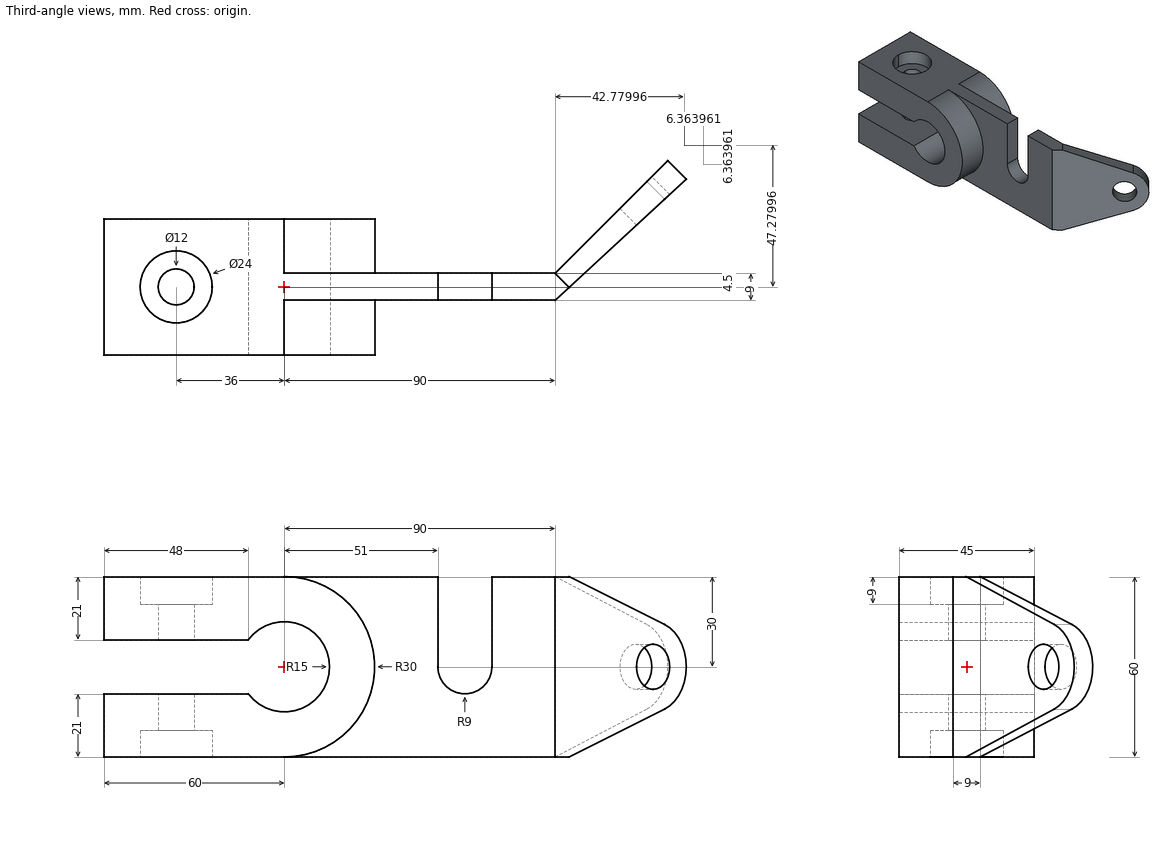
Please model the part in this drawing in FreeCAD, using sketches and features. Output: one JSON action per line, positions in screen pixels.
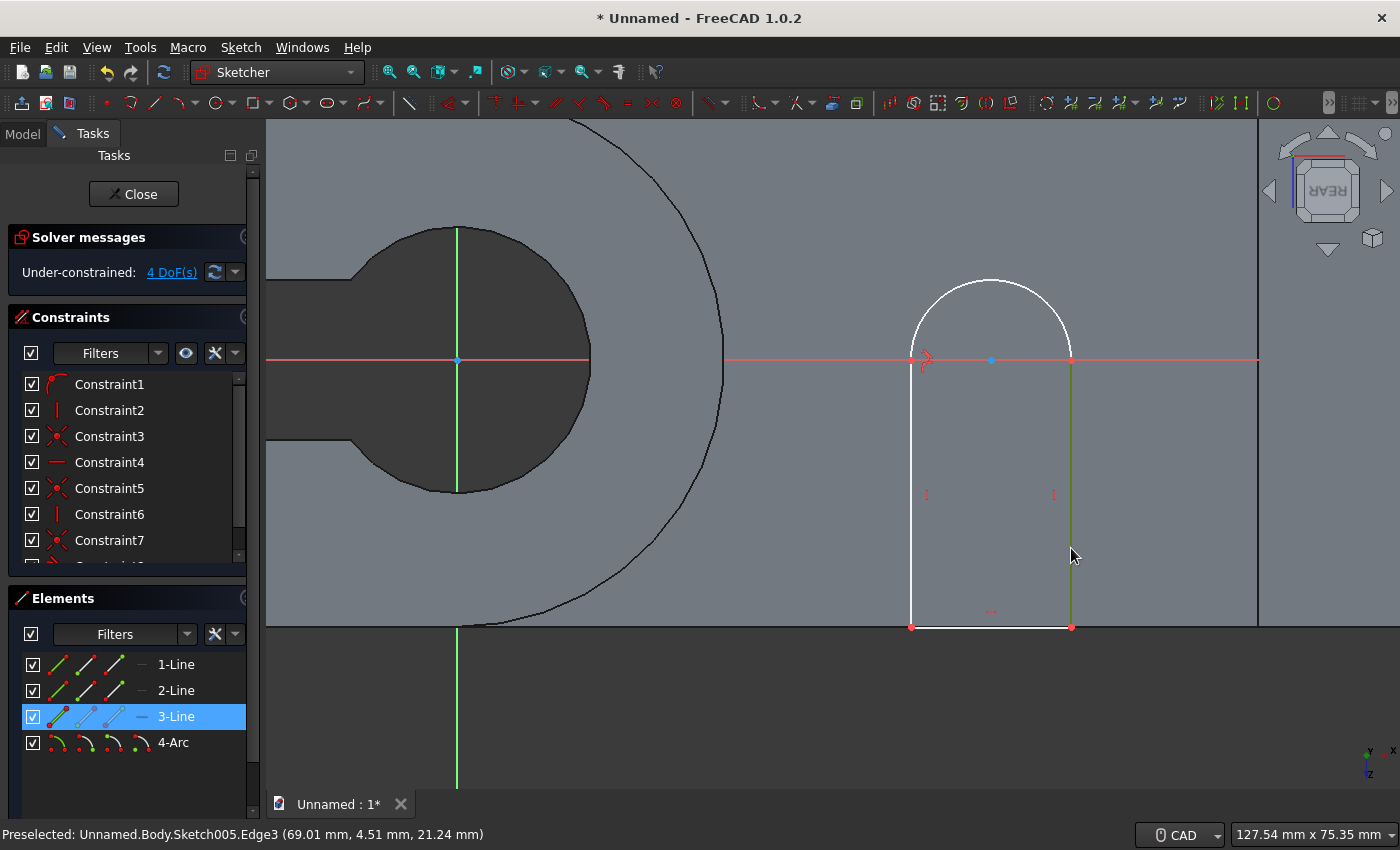
{"action": "left_click", "coordinate": [1039, 296]}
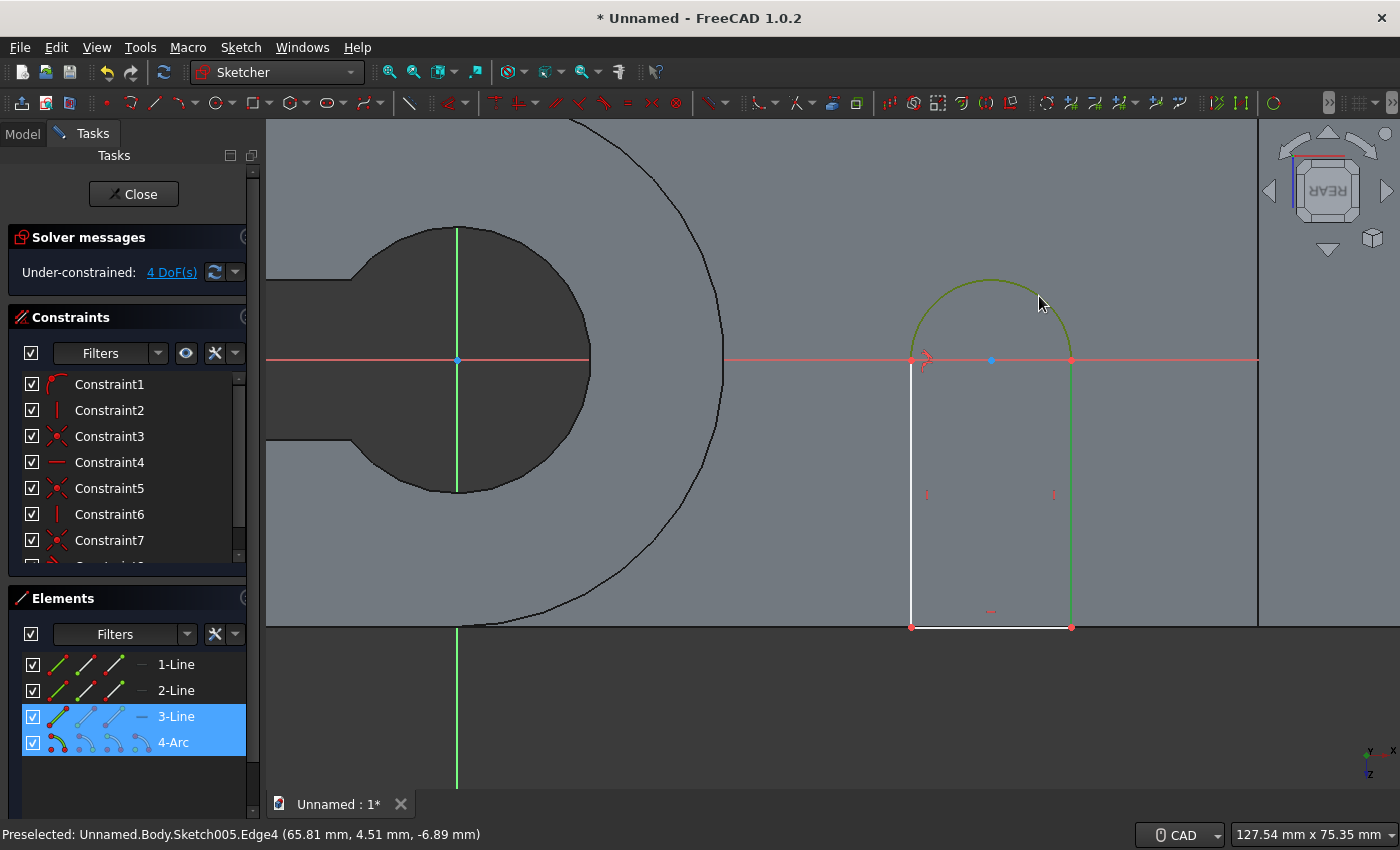
{"action": "key", "text": "t"}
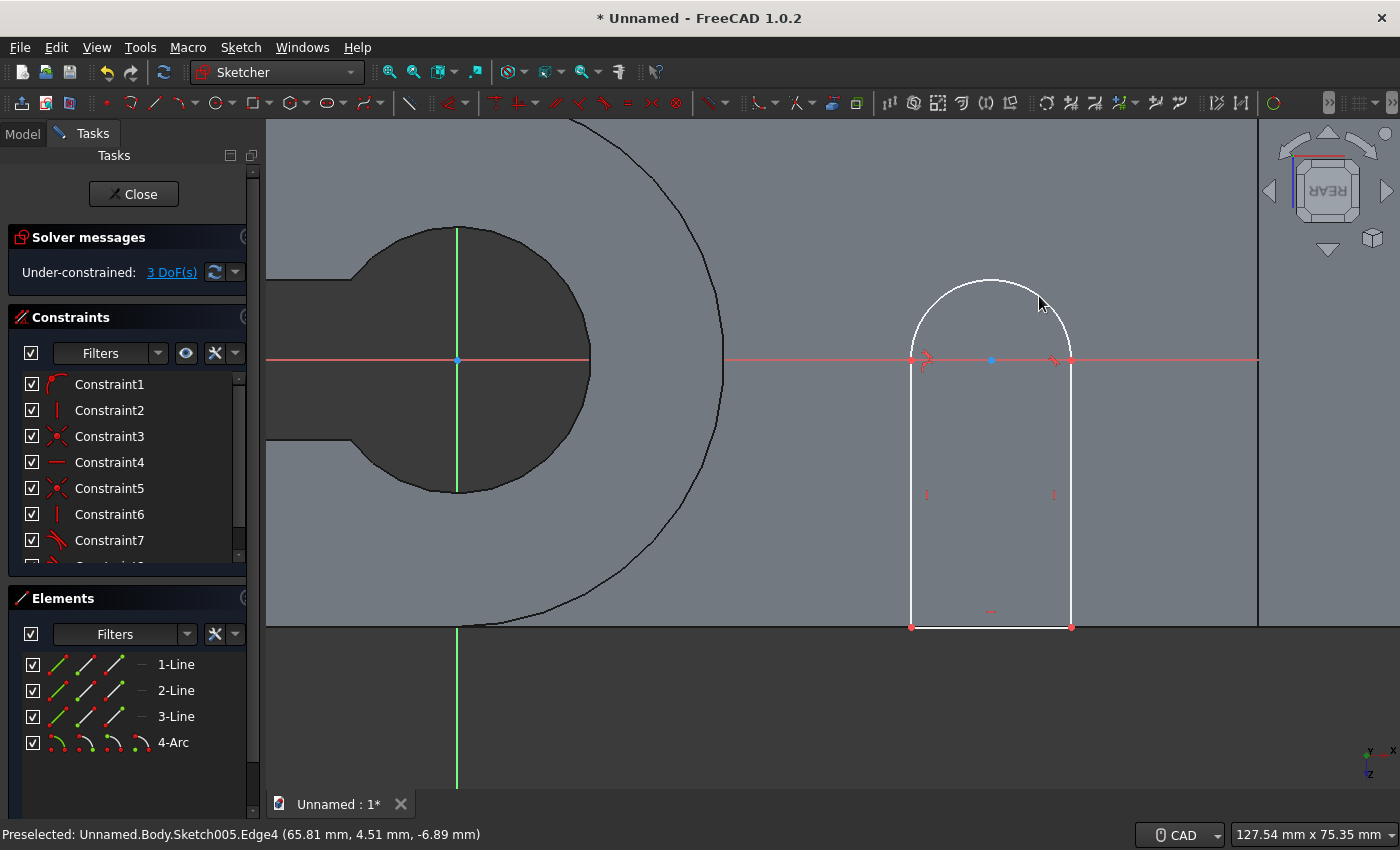
{"action": "key", "text": "d"}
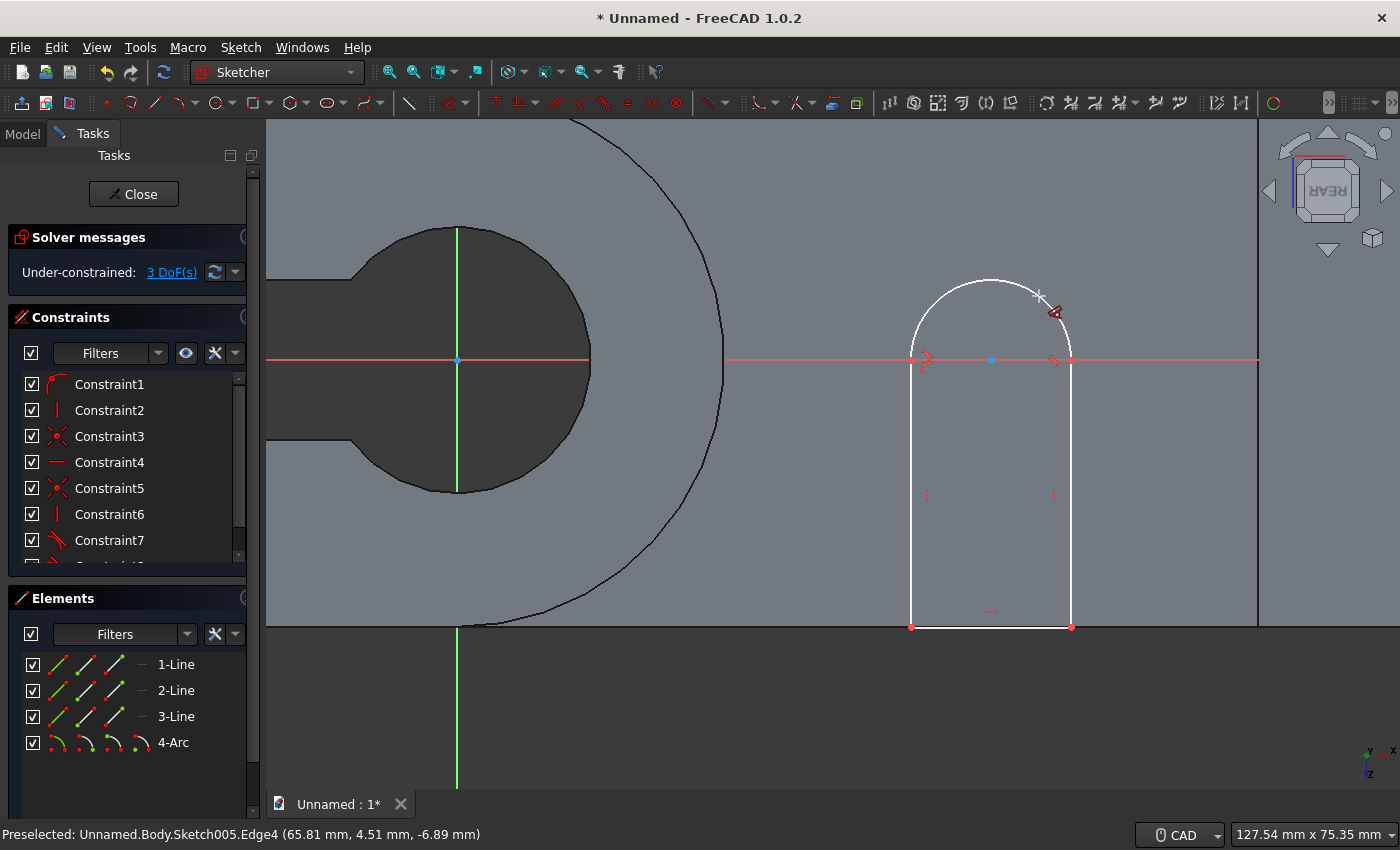
{"action": "left_click", "coordinate": [1038, 295]}
{"action": "left_click", "coordinate": [1057, 269]}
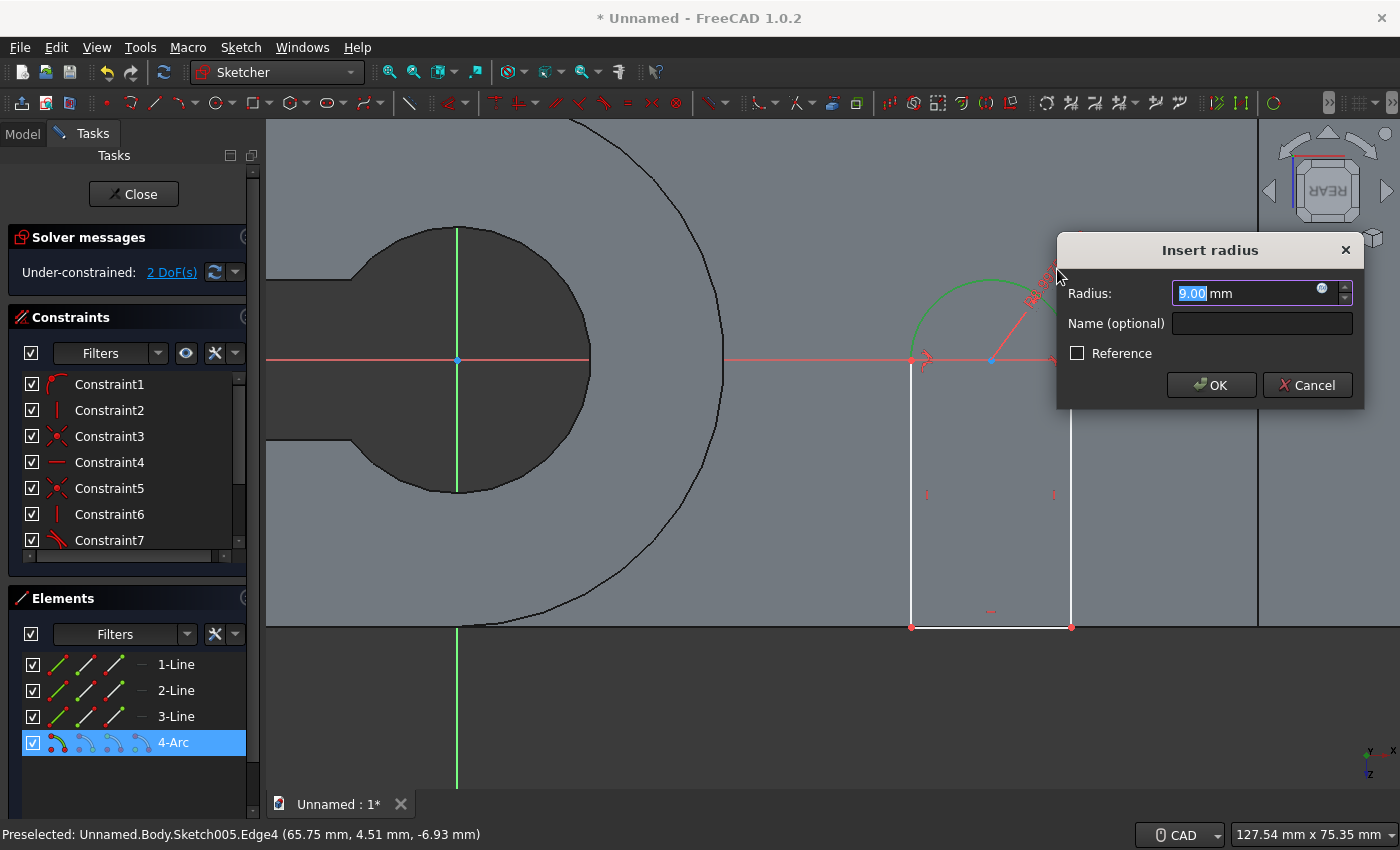
{"action": "type", "text": "9"}
{"action": "key", "text": "Return"}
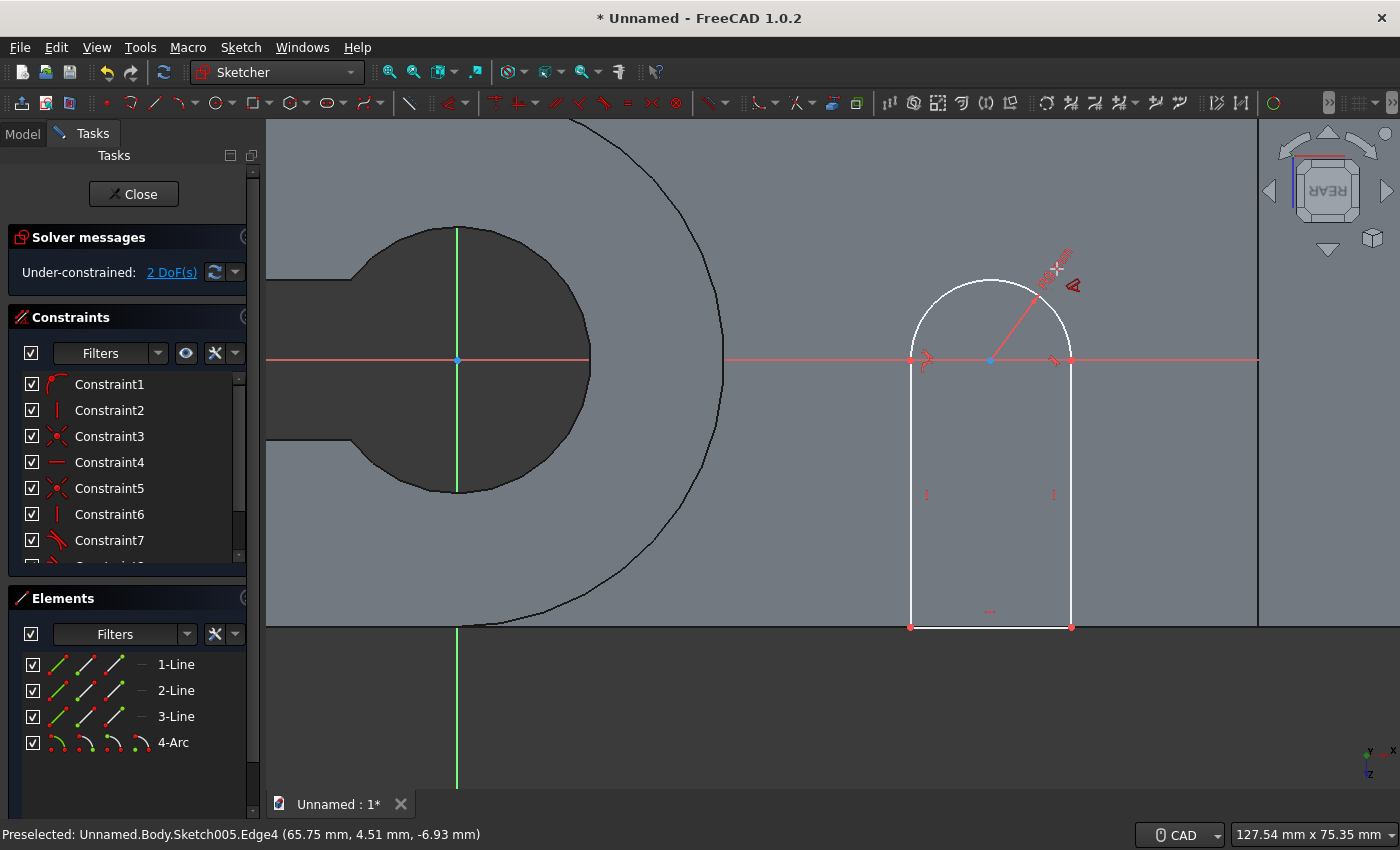
{"action": "left_click", "coordinate": [911, 440]}
{"action": "left_click", "coordinate": [945, 494]}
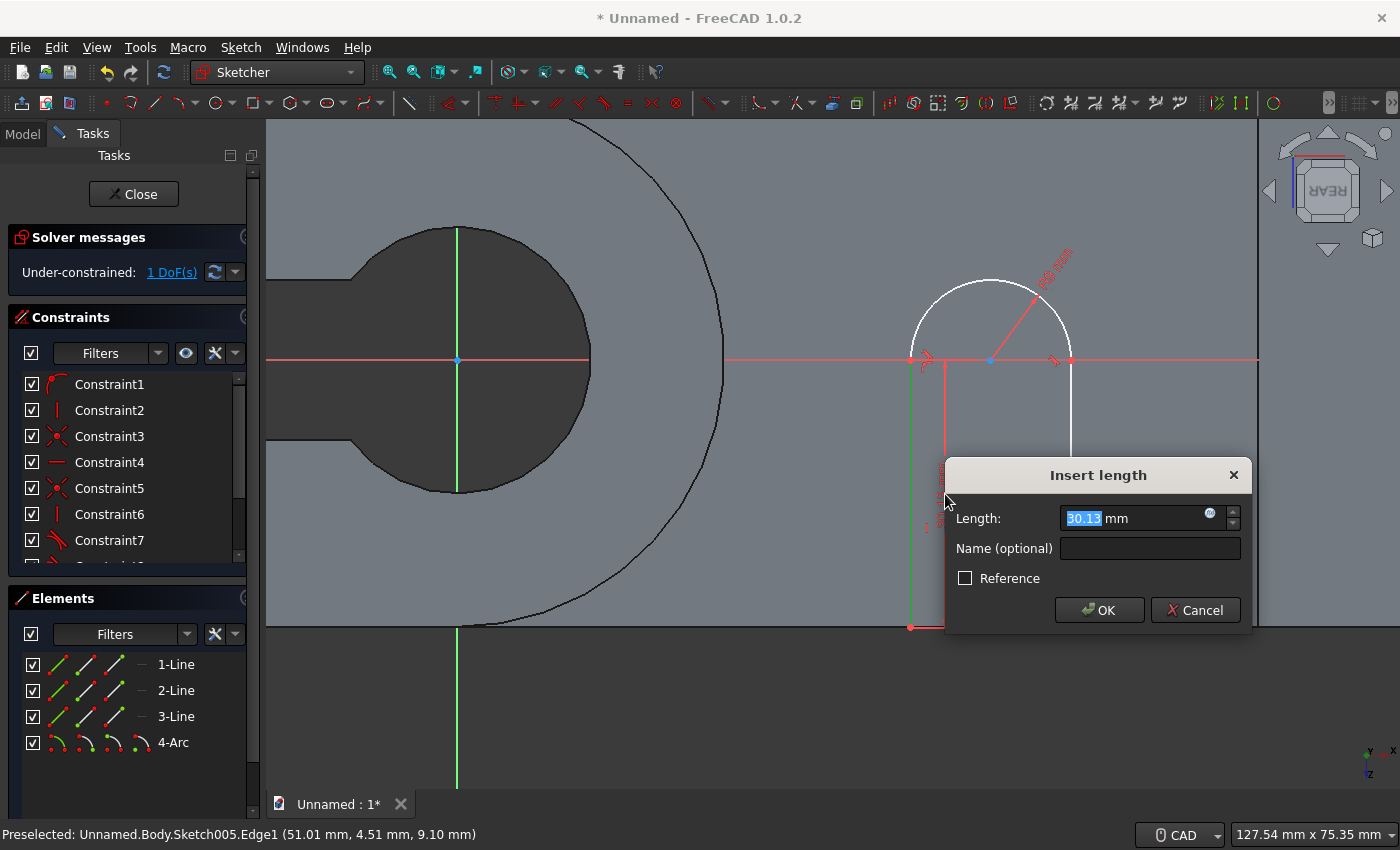
{"action": "type", "text": "30"}
{"action": "key", "text": "Return"}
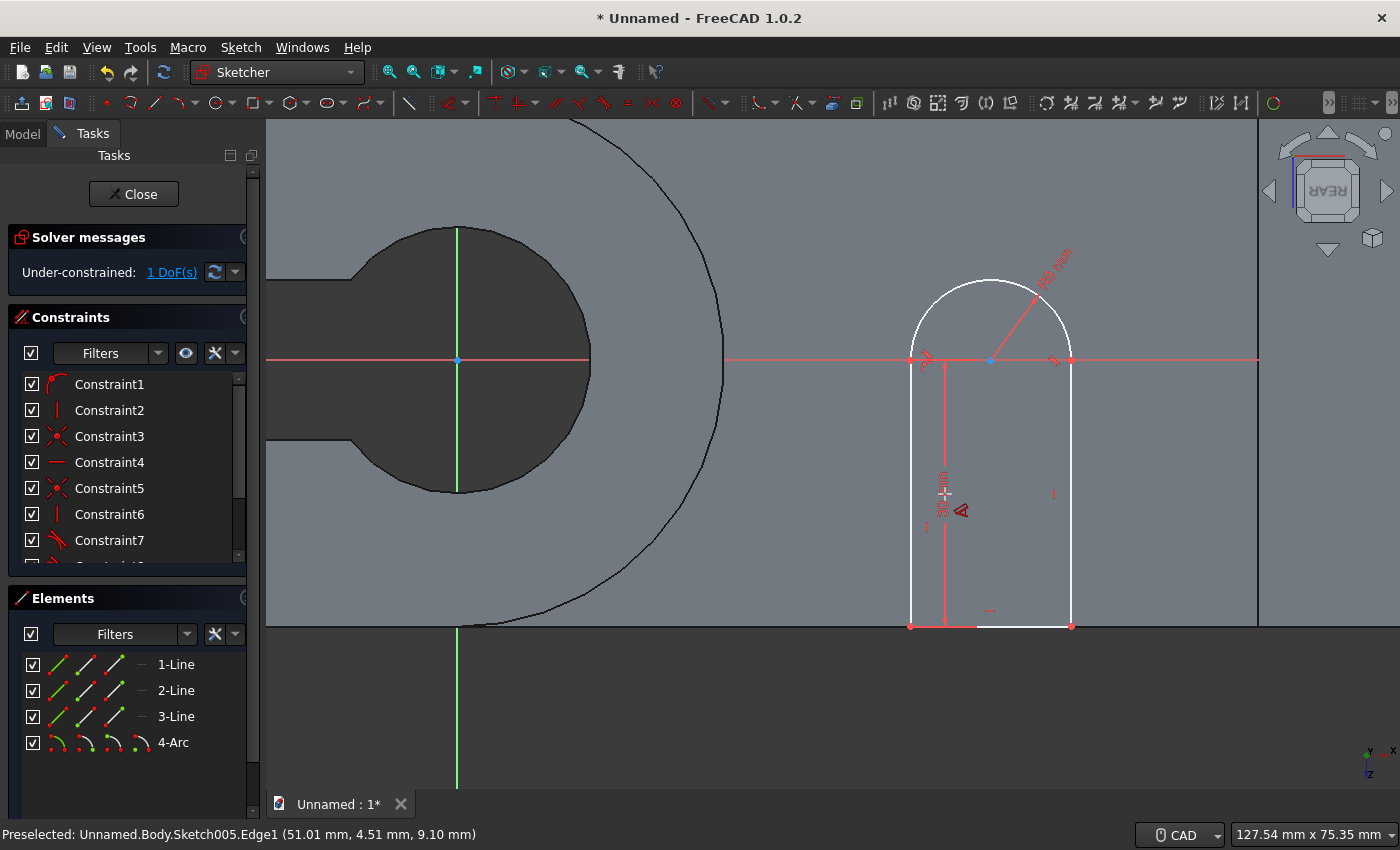
{"action": "left_click", "coordinate": [911, 360]}
{"action": "left_click", "coordinate": [684, 326]}